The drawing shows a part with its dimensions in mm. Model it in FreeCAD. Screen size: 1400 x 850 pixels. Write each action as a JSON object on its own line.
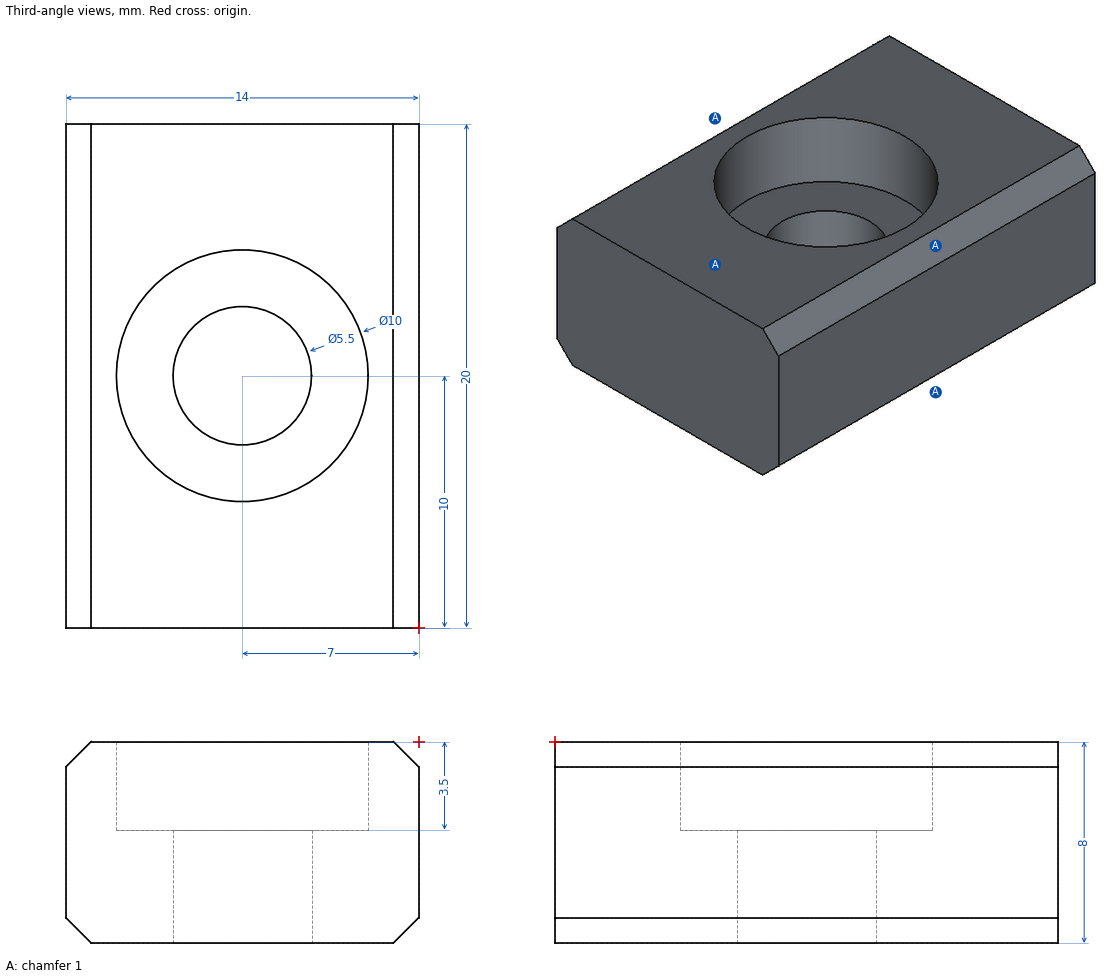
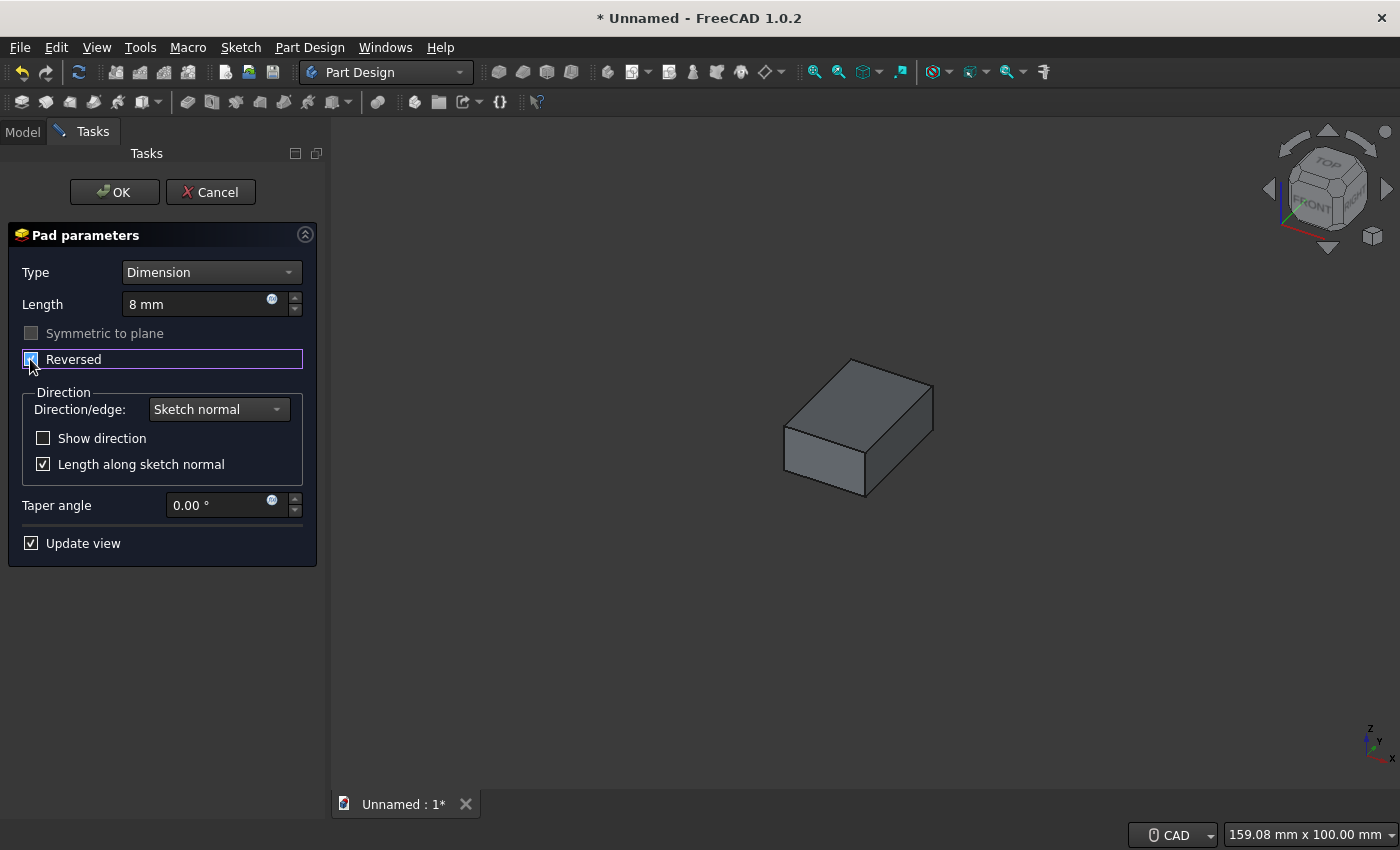
{"action": "left_click", "coordinate": [115, 192]}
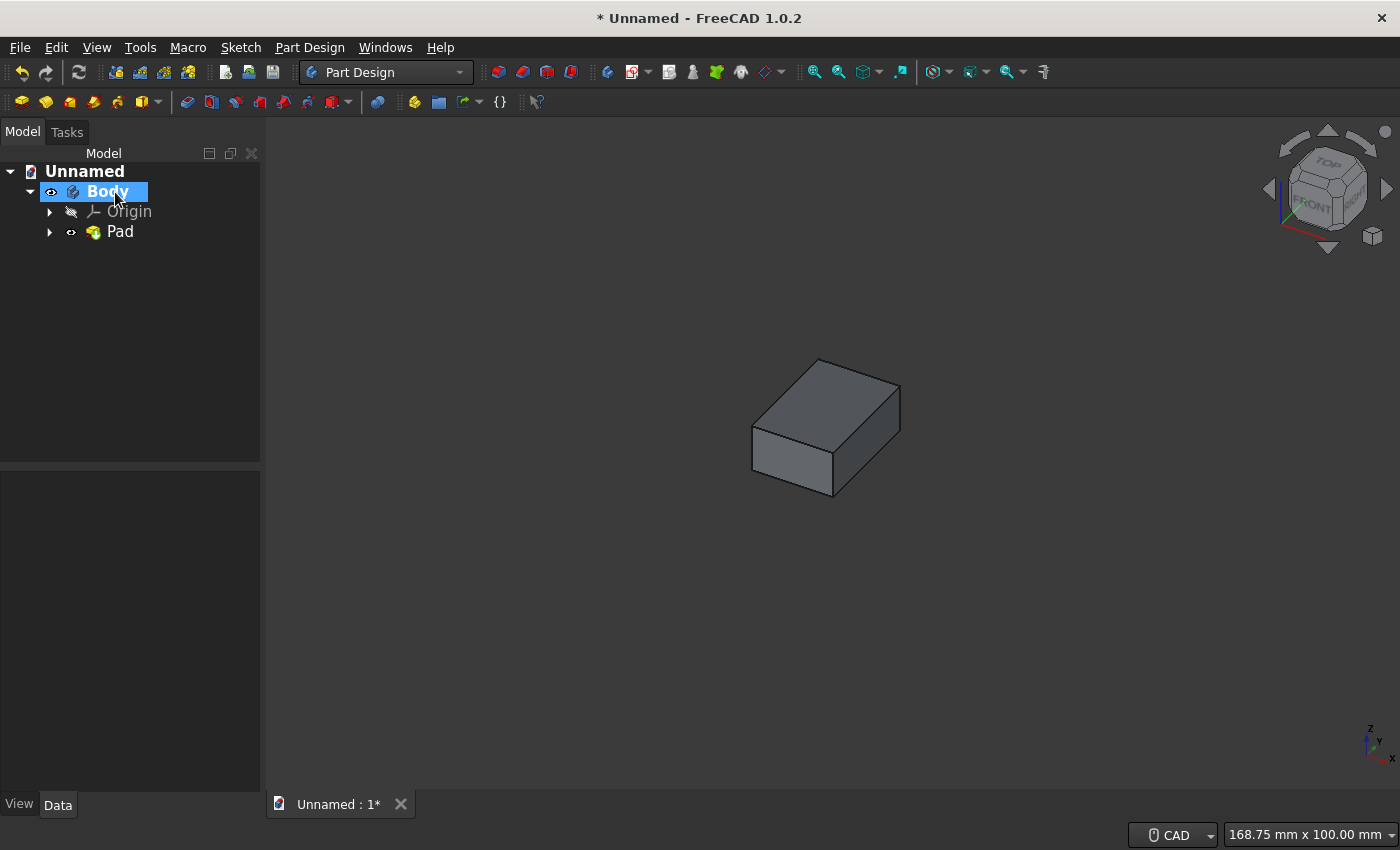
{"action": "key", "text": "v f"}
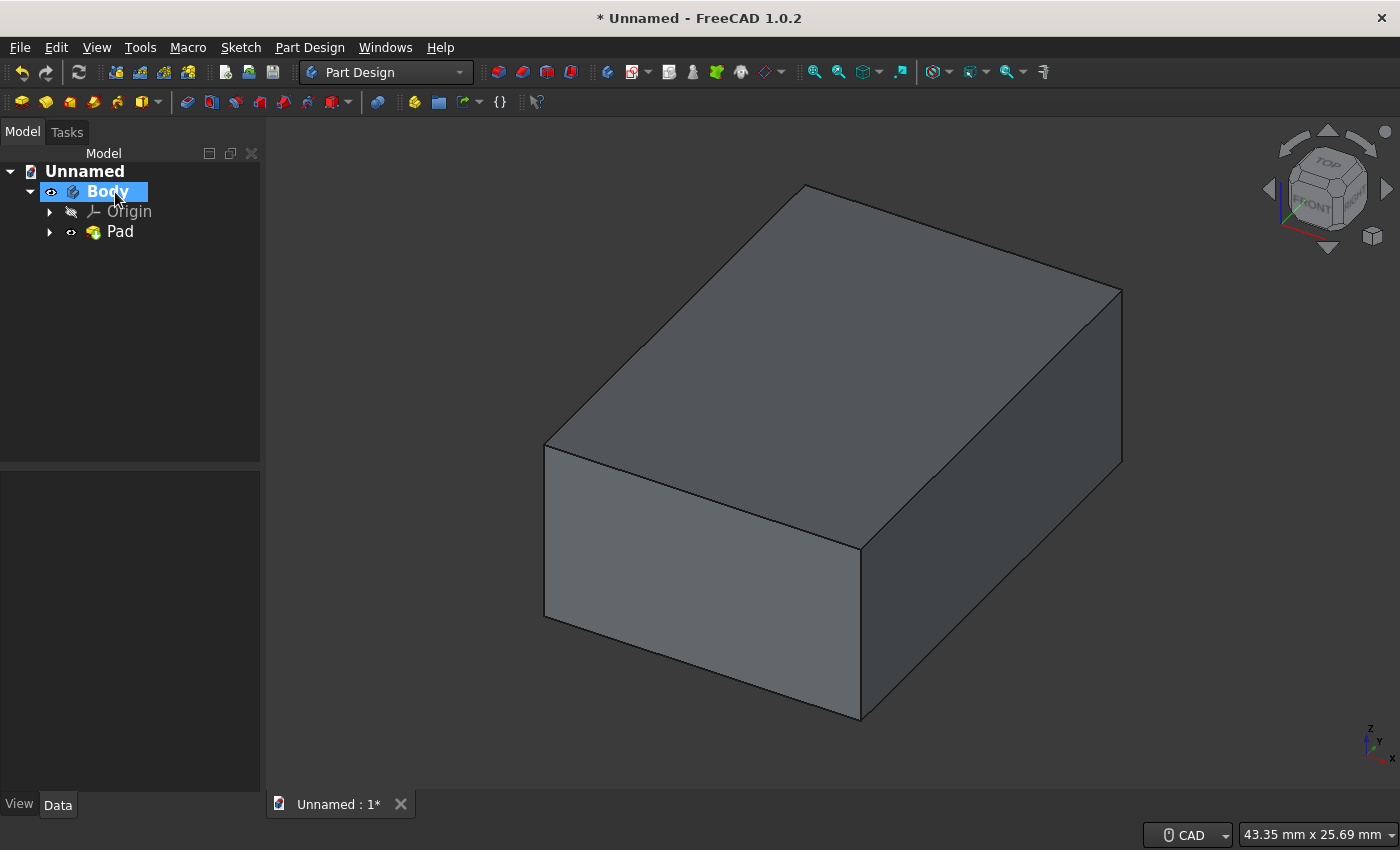
{"action": "left_click", "coordinate": [632, 72]}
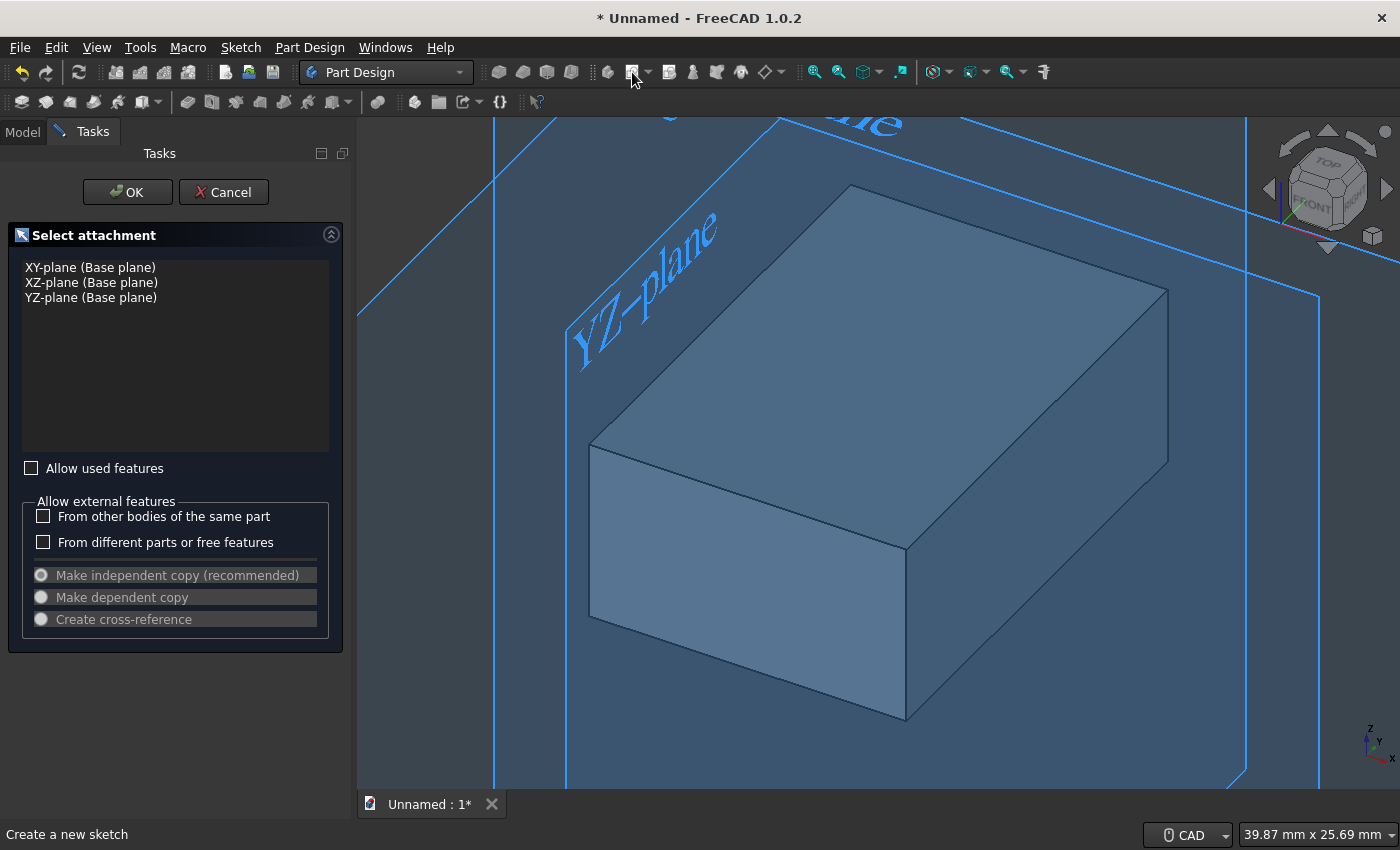
{"action": "left_click", "coordinate": [82, 268]}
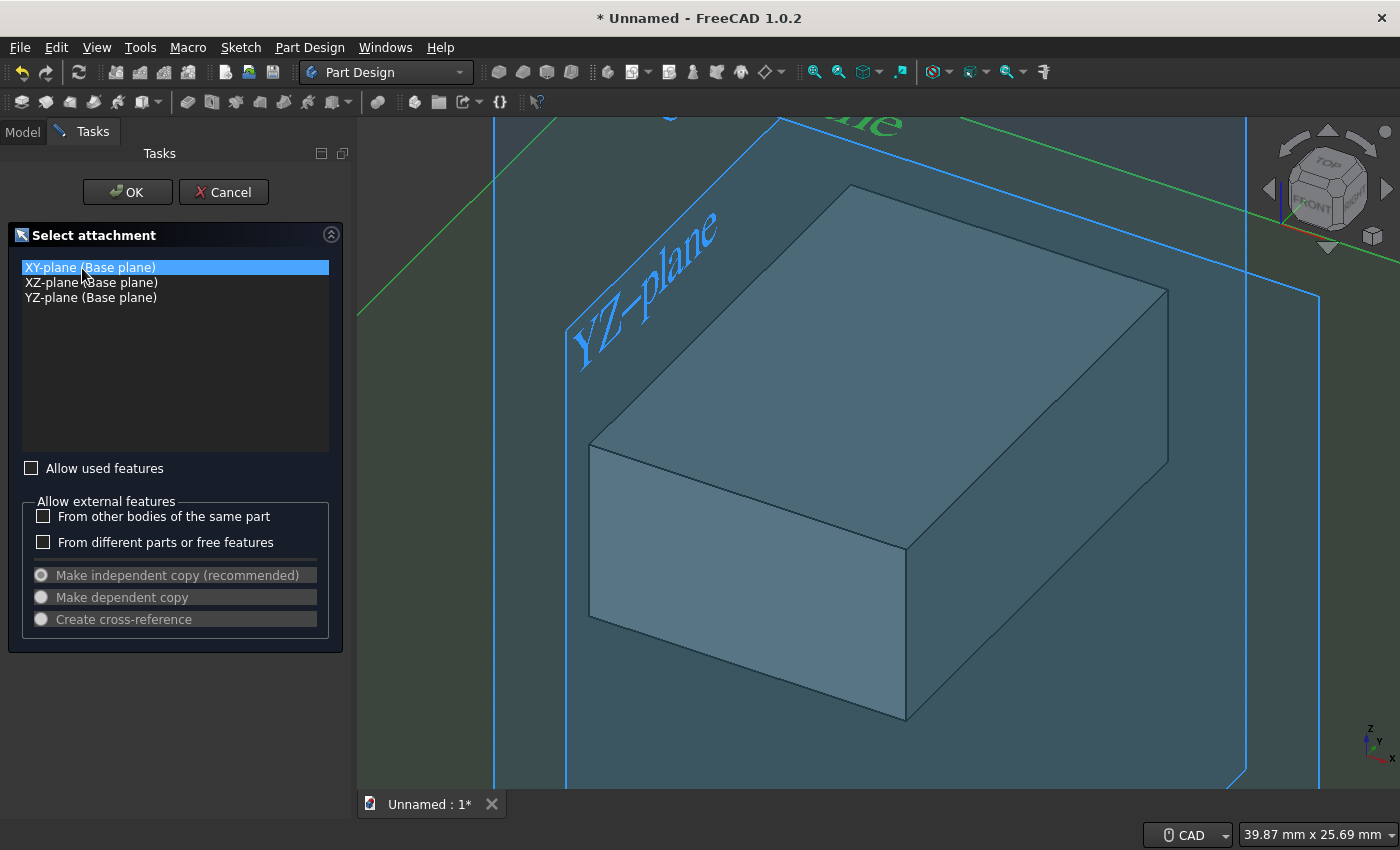
{"action": "left_click", "coordinate": [128, 192]}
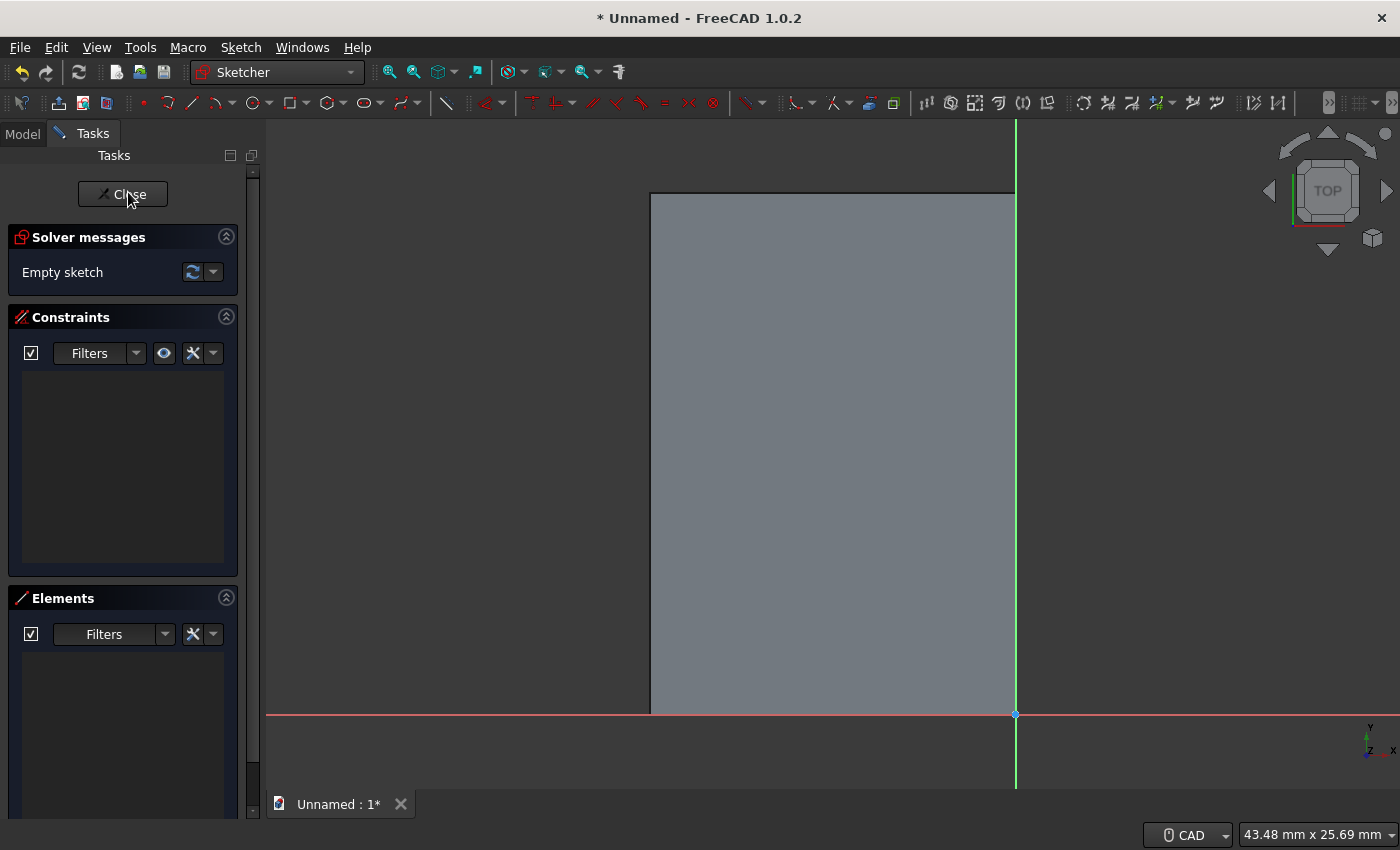
{"action": "left_click", "coordinate": [254, 104]}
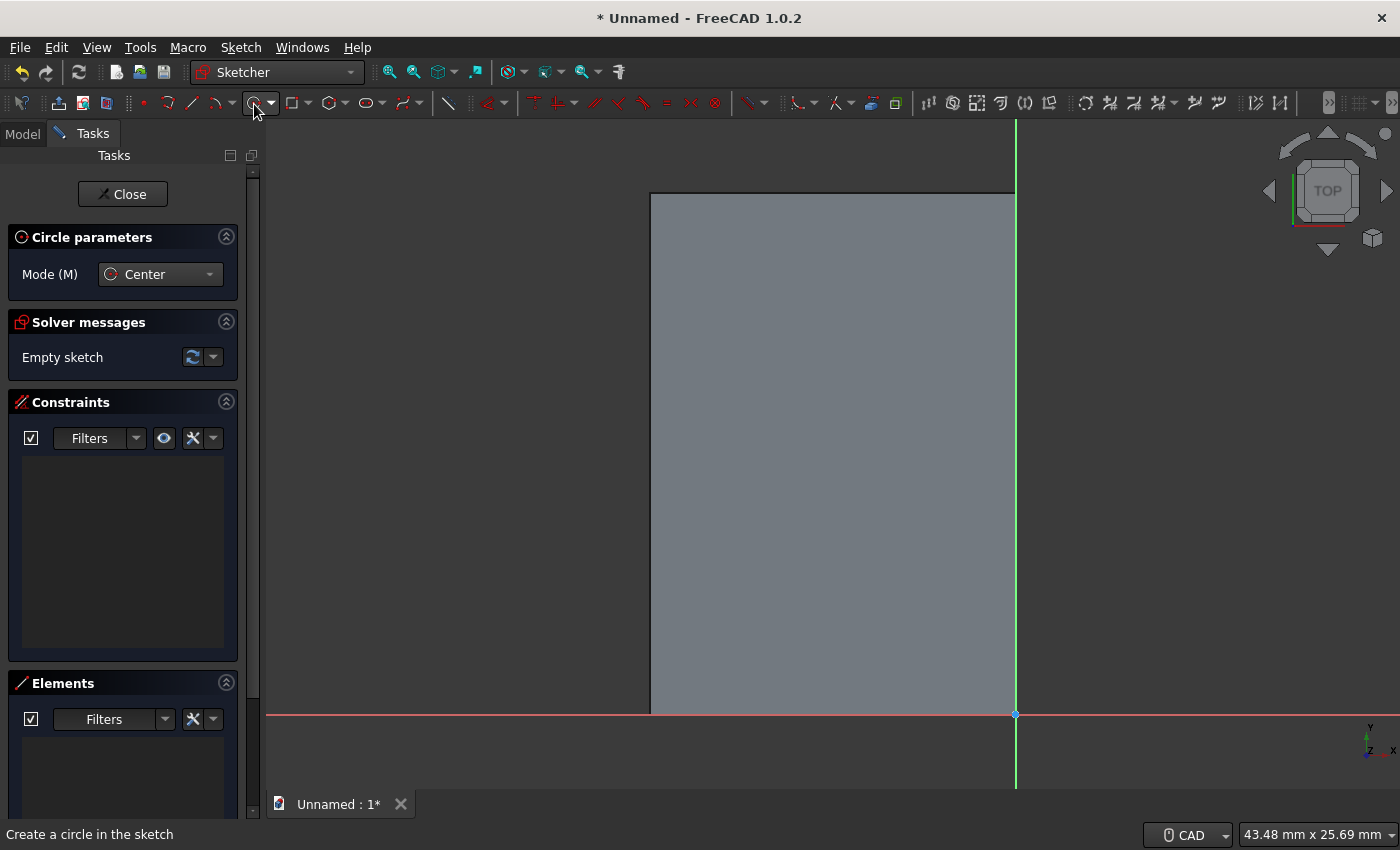
{"action": "left_click", "coordinate": [833, 454]}
{"action": "left_click", "coordinate": [925, 362]}
{"action": "key", "text": "Escape"}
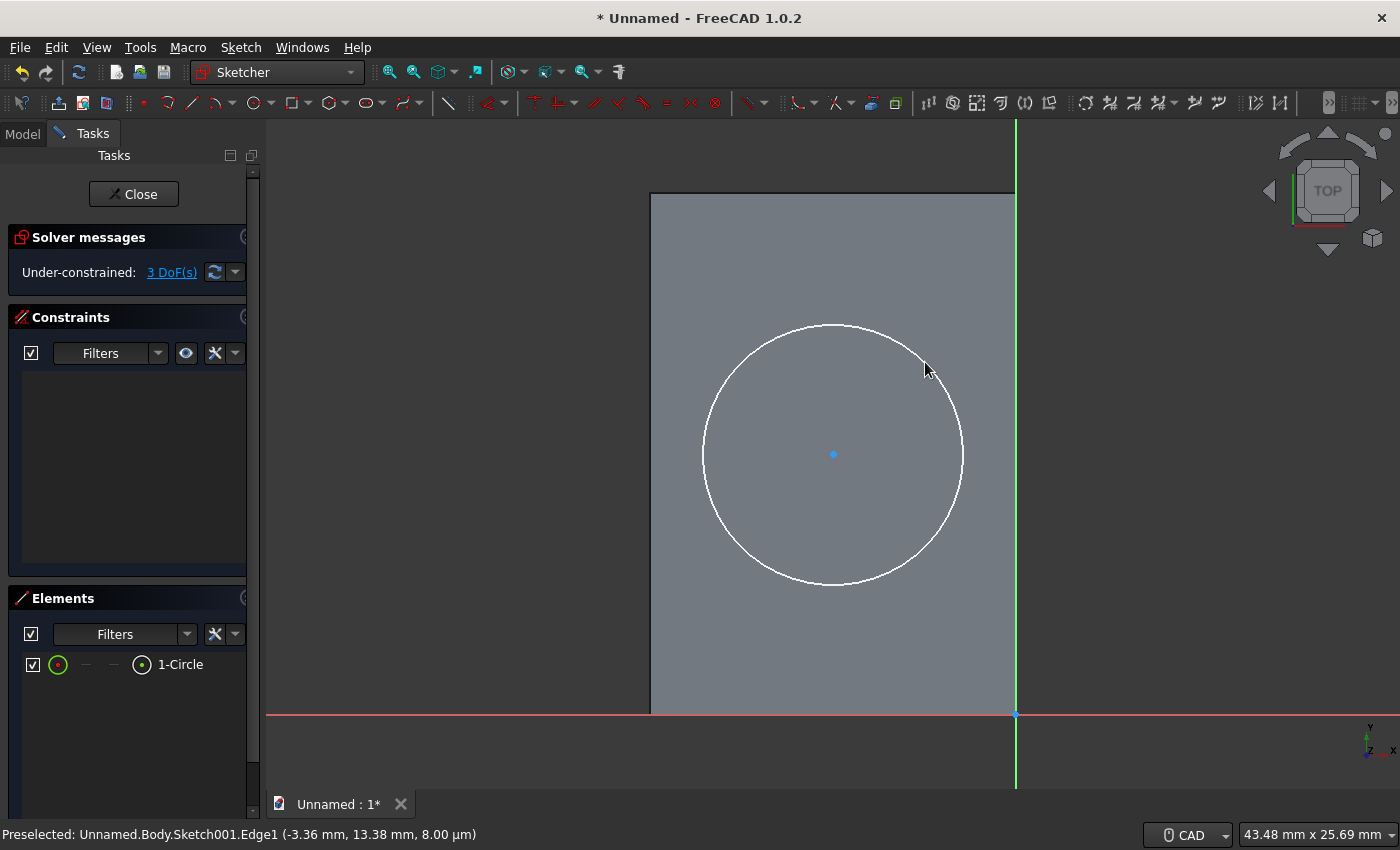
{"action": "key", "text": "d"}